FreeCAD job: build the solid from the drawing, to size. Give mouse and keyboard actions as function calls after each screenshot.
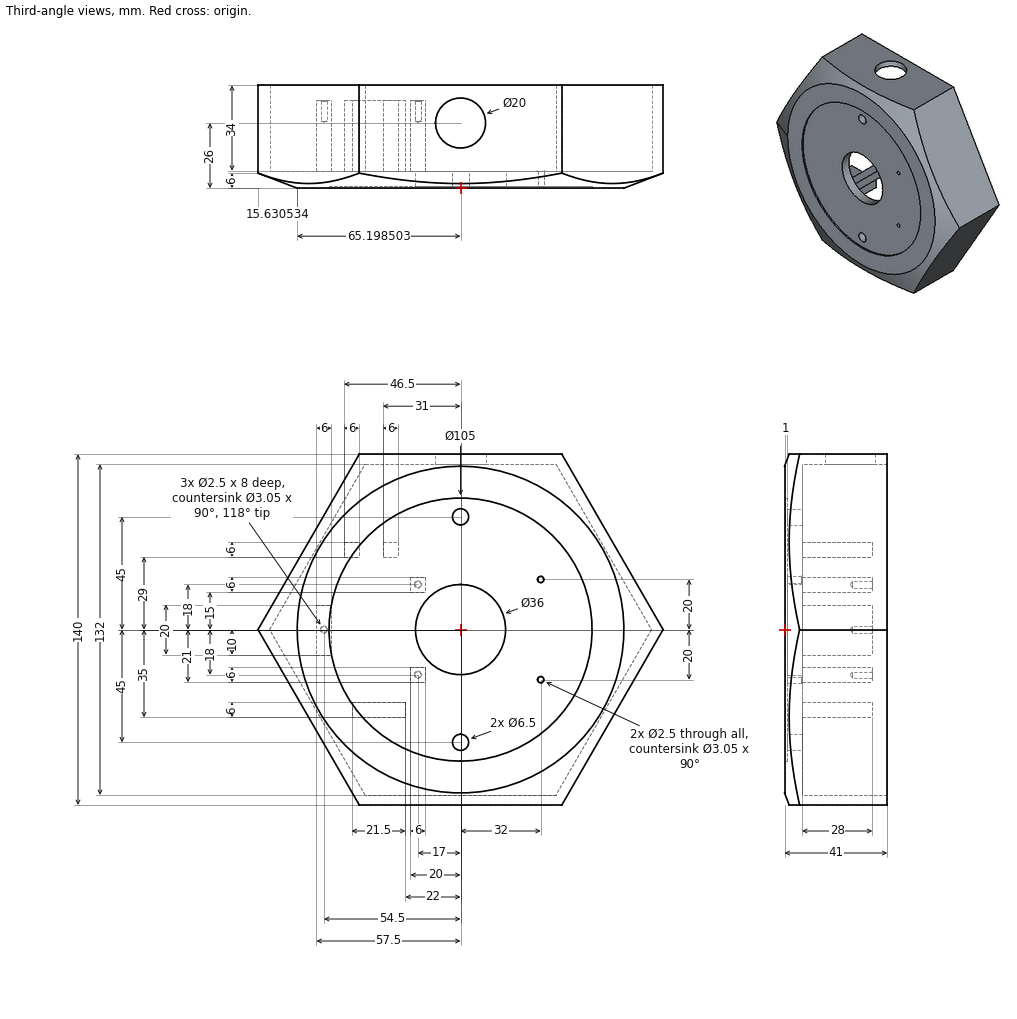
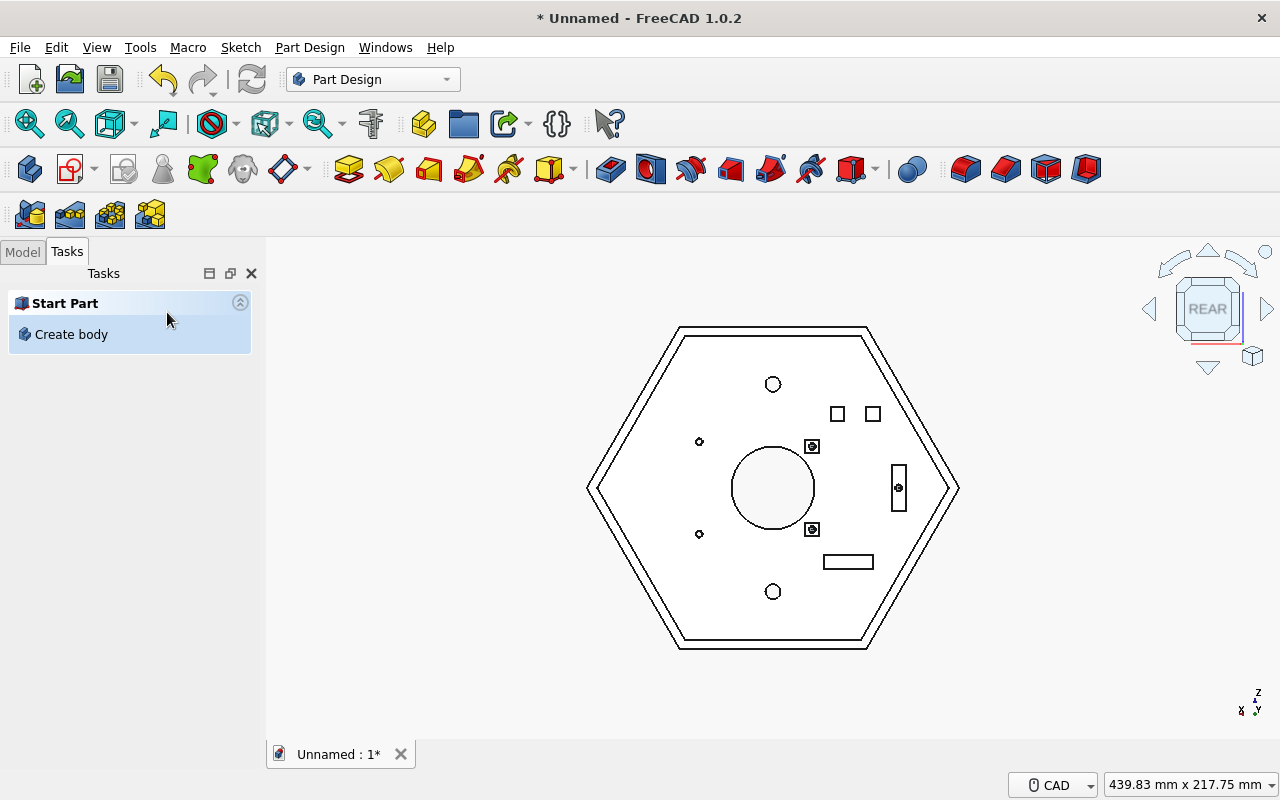
click(23, 251)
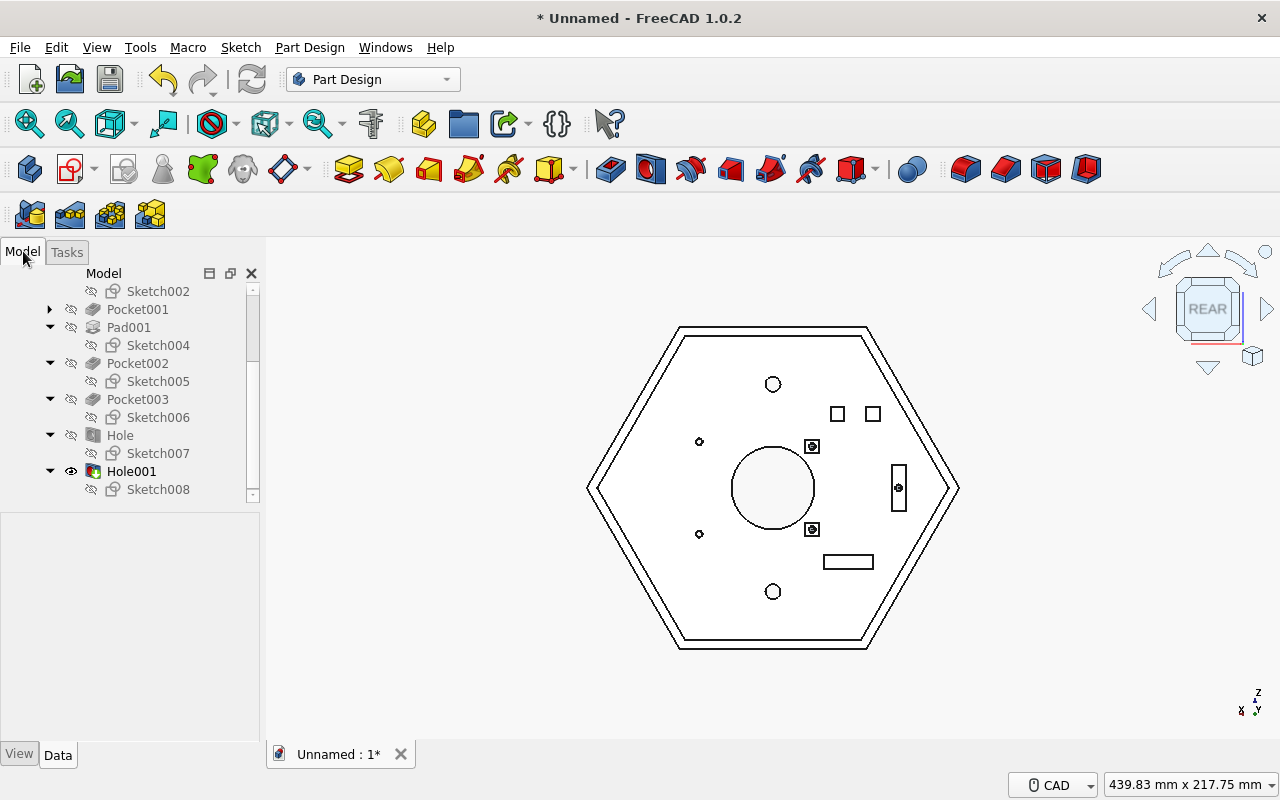
scroll(160, 395, down, 3)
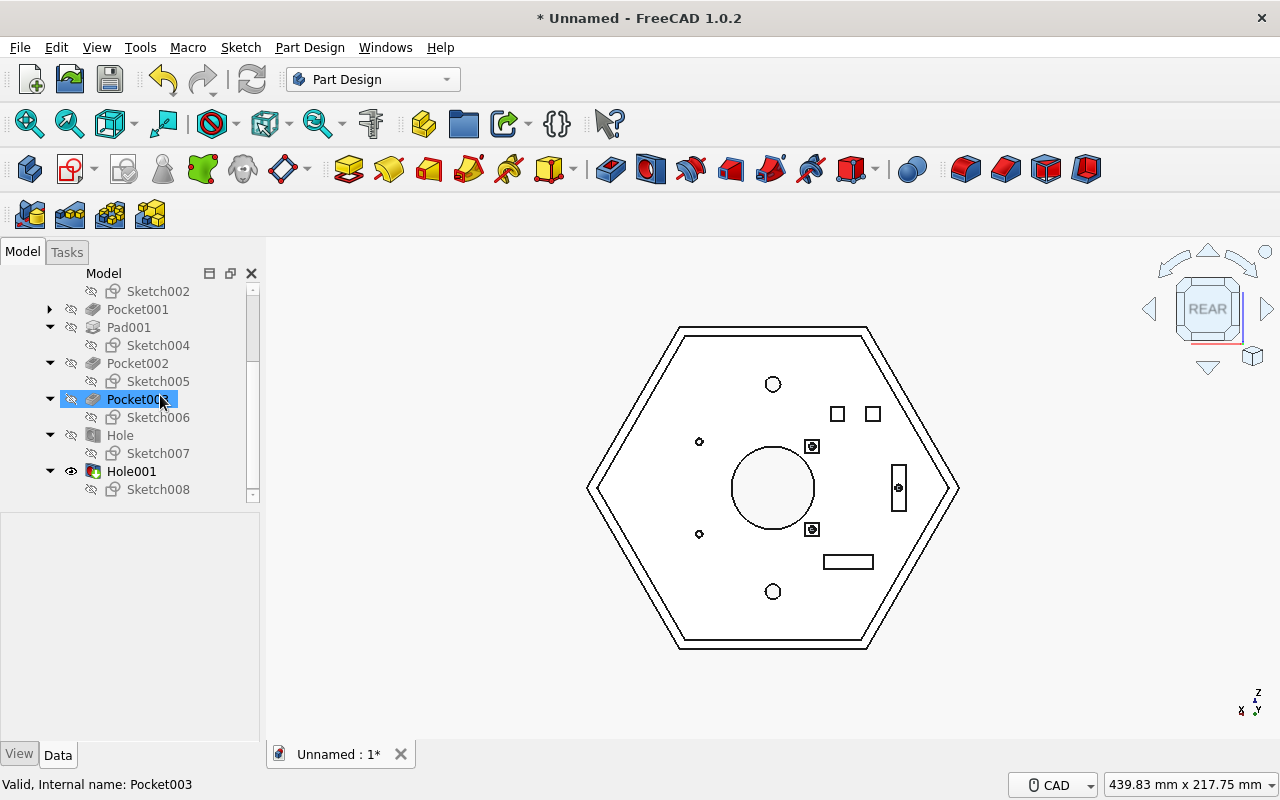
scroll(160, 395, up, 15)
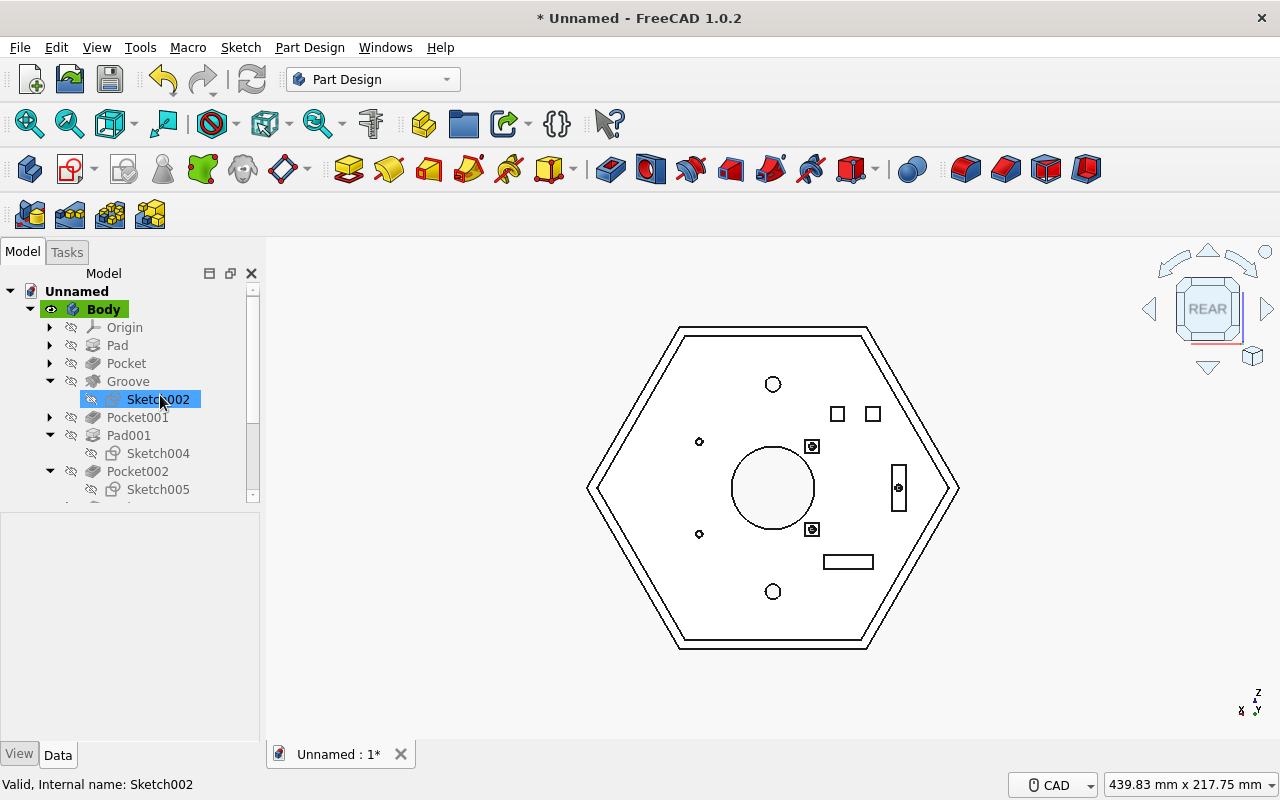
click(50, 327)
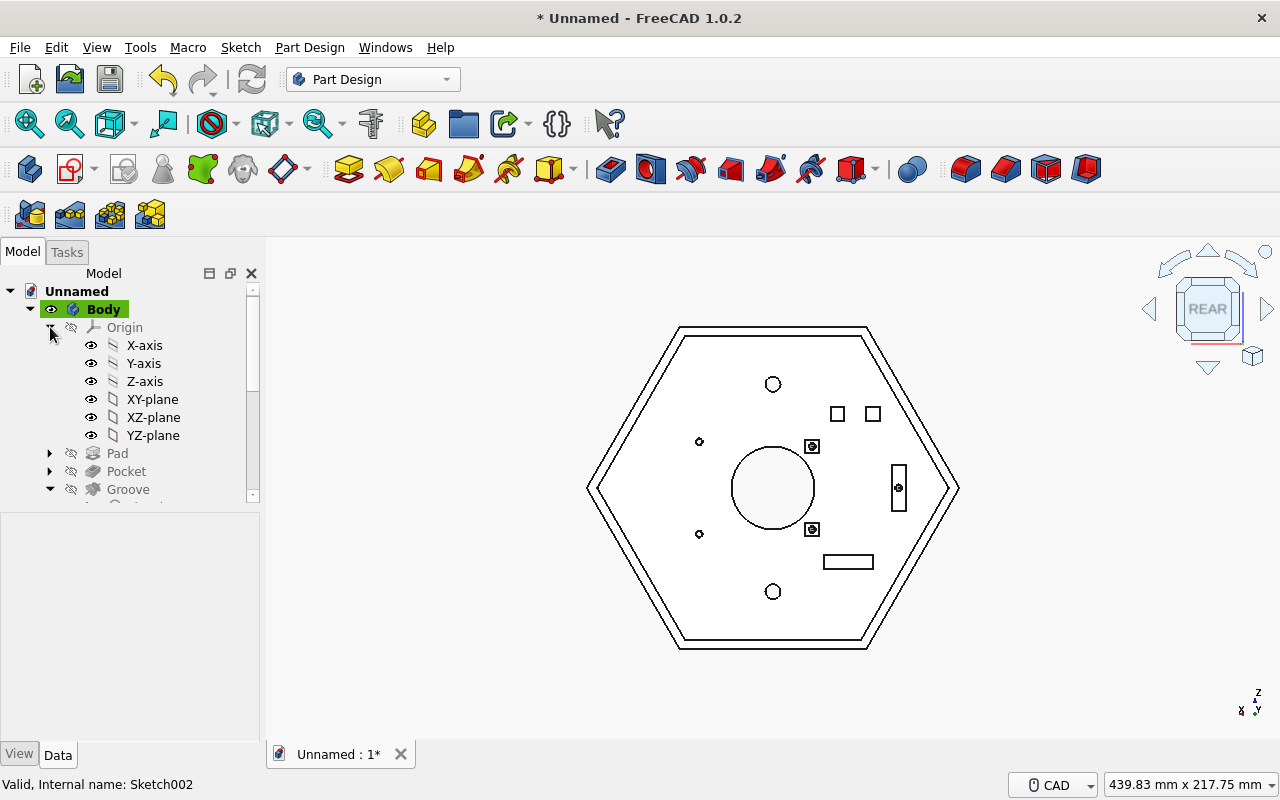
click(136, 399)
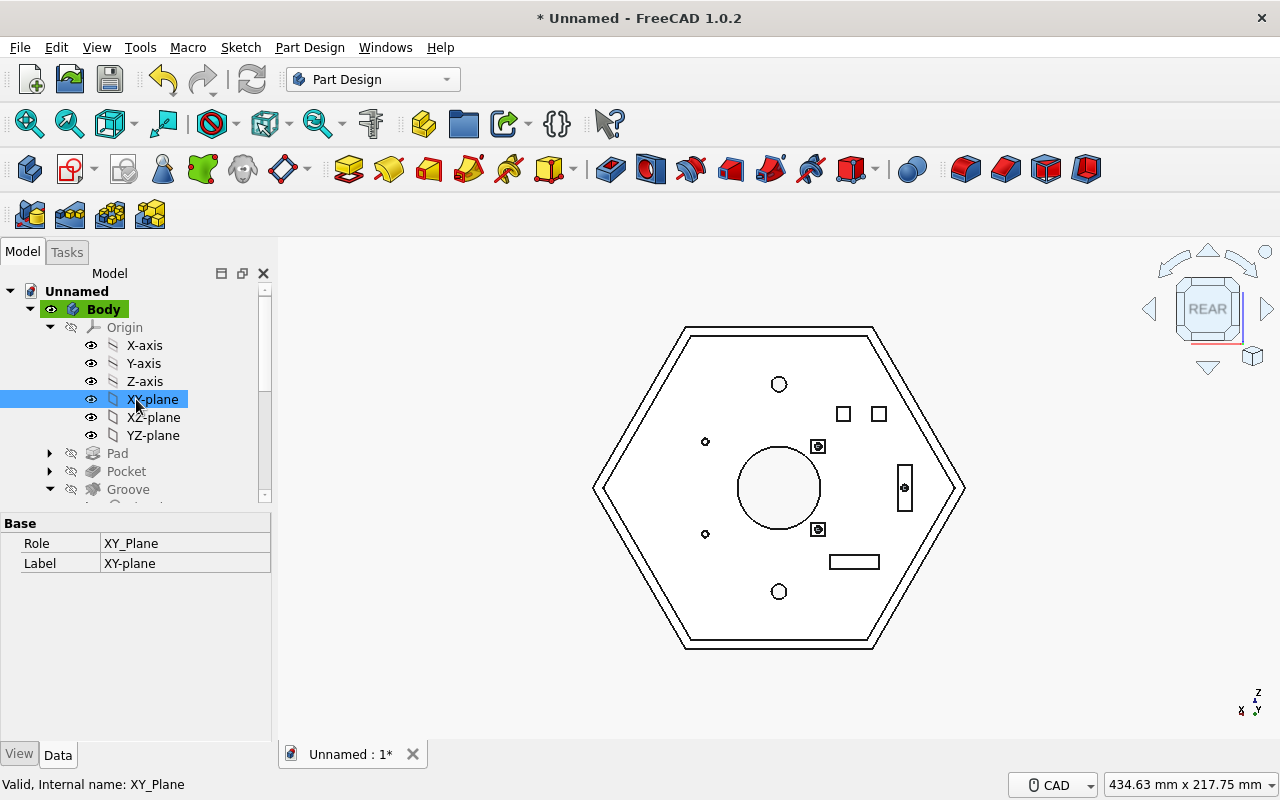
click(284, 170)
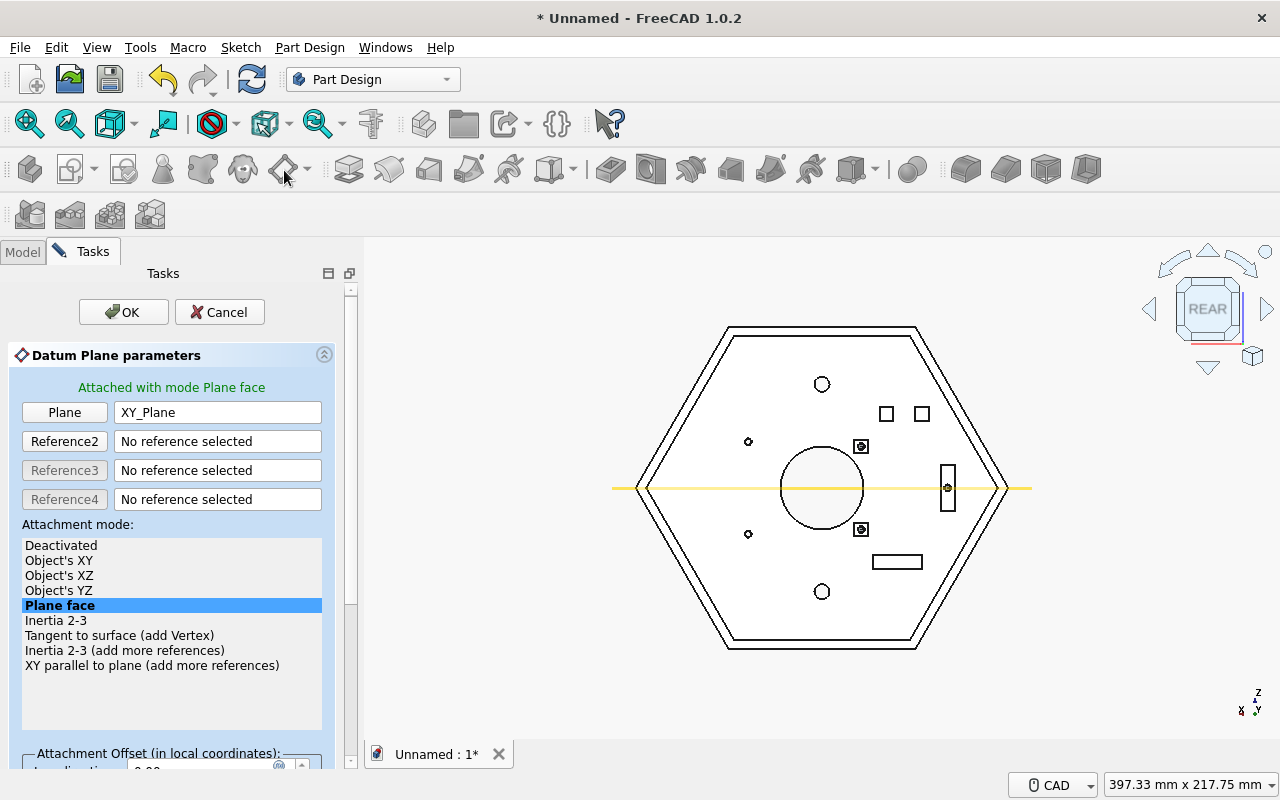
scroll(351, 526, down, 3)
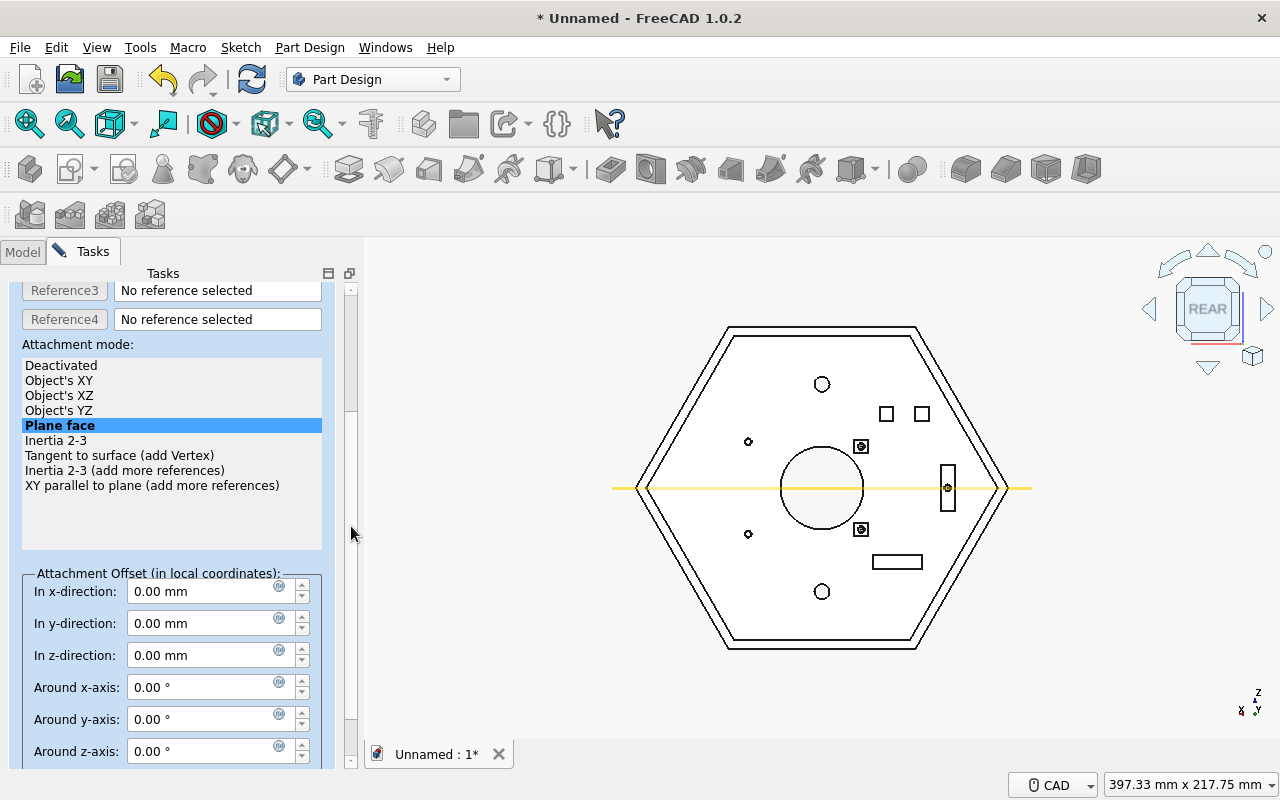
triple_click(210, 655)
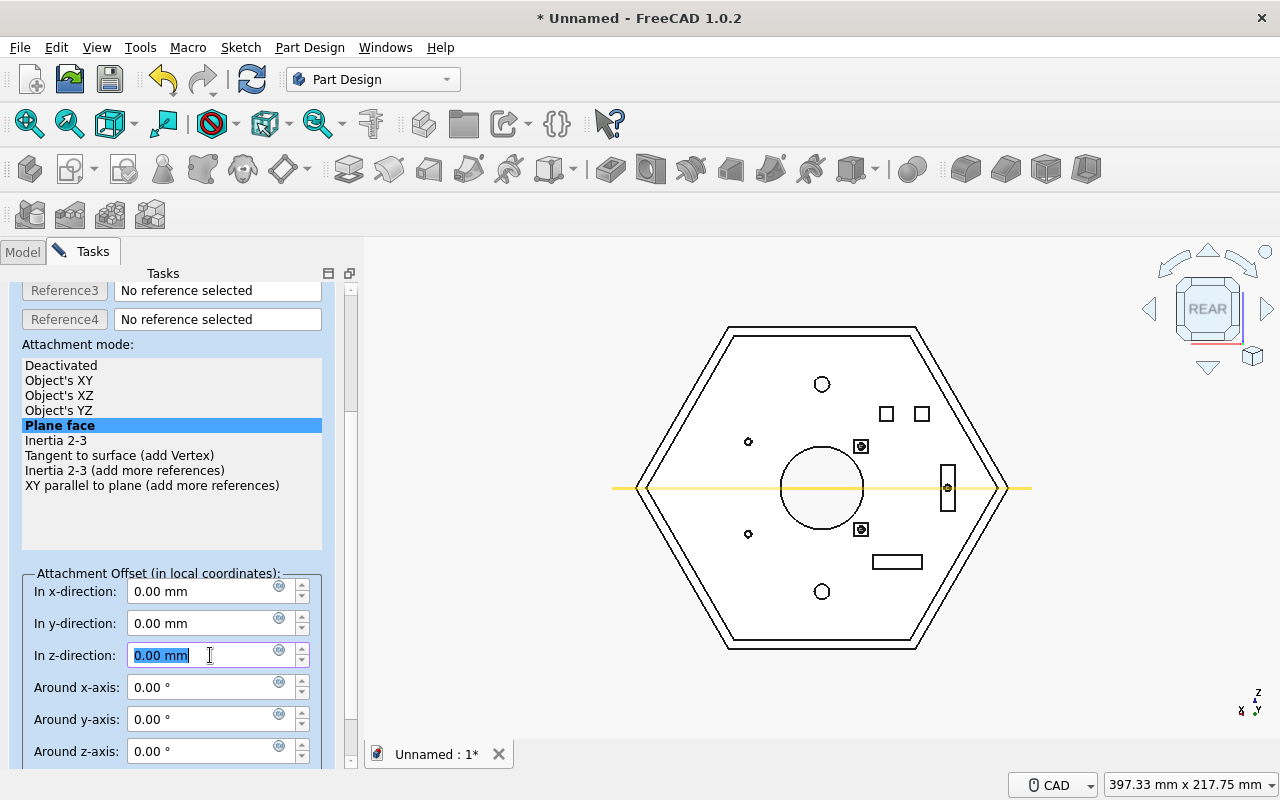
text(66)
key(Tab)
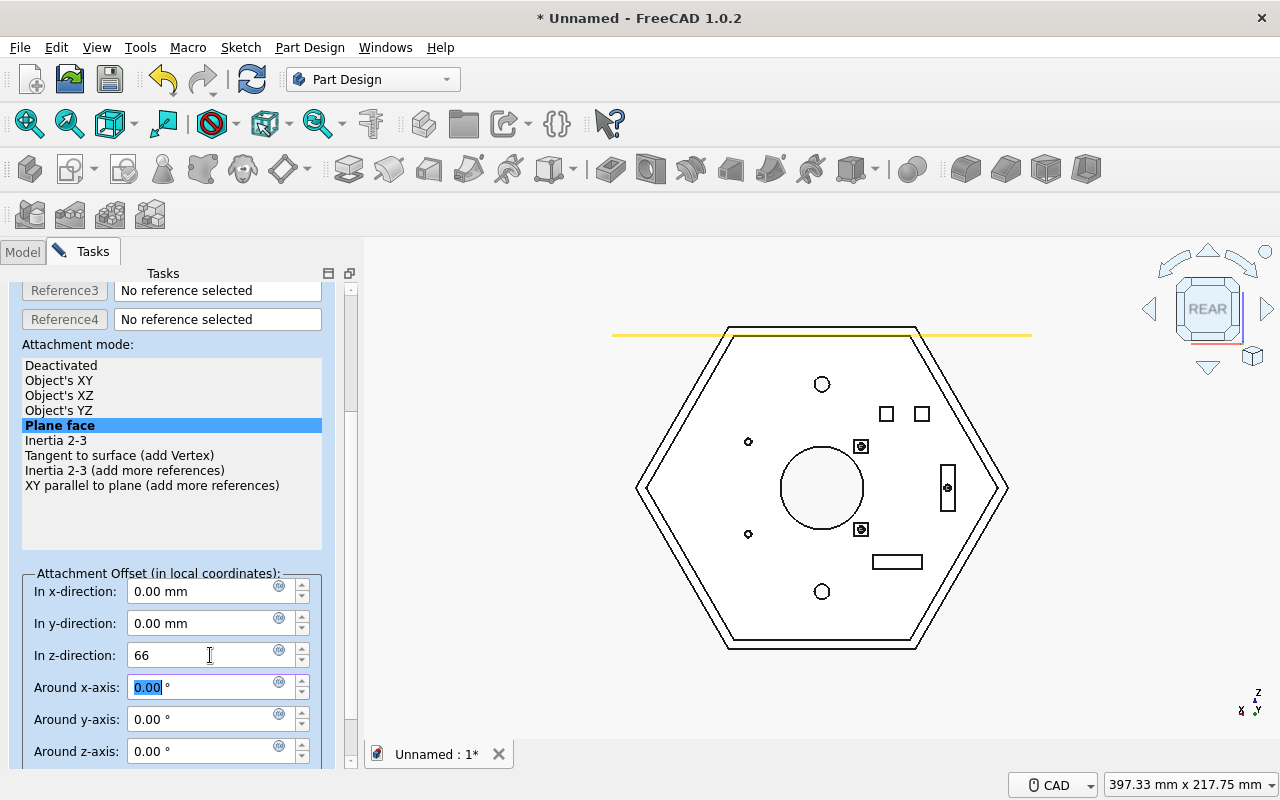
scroll(351, 526, up, 4)